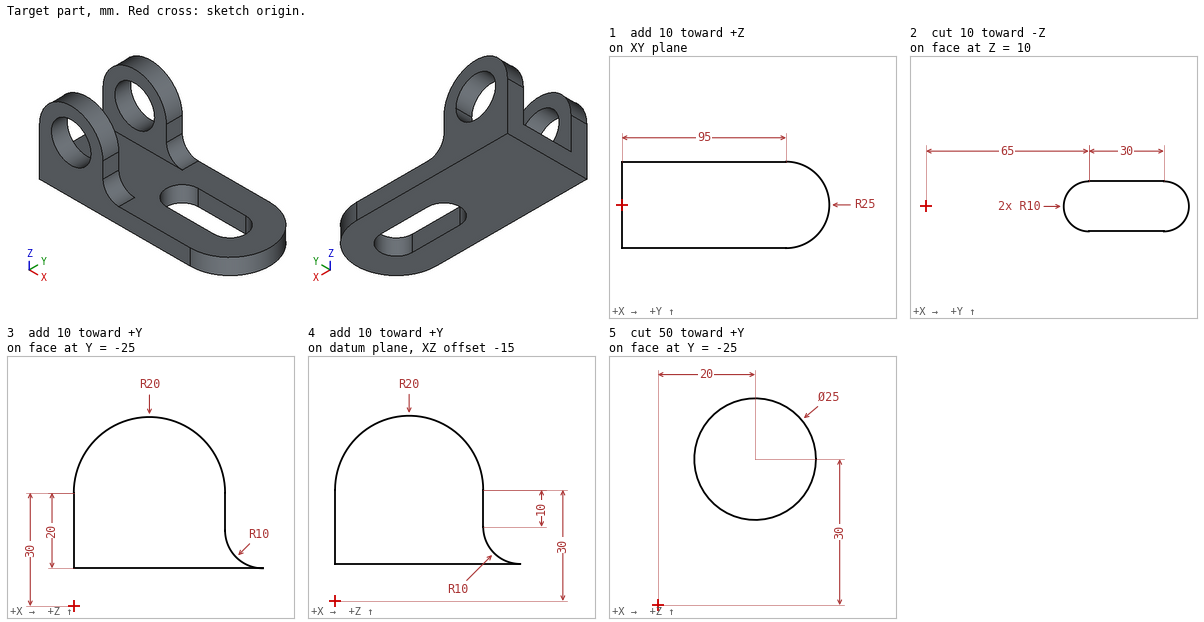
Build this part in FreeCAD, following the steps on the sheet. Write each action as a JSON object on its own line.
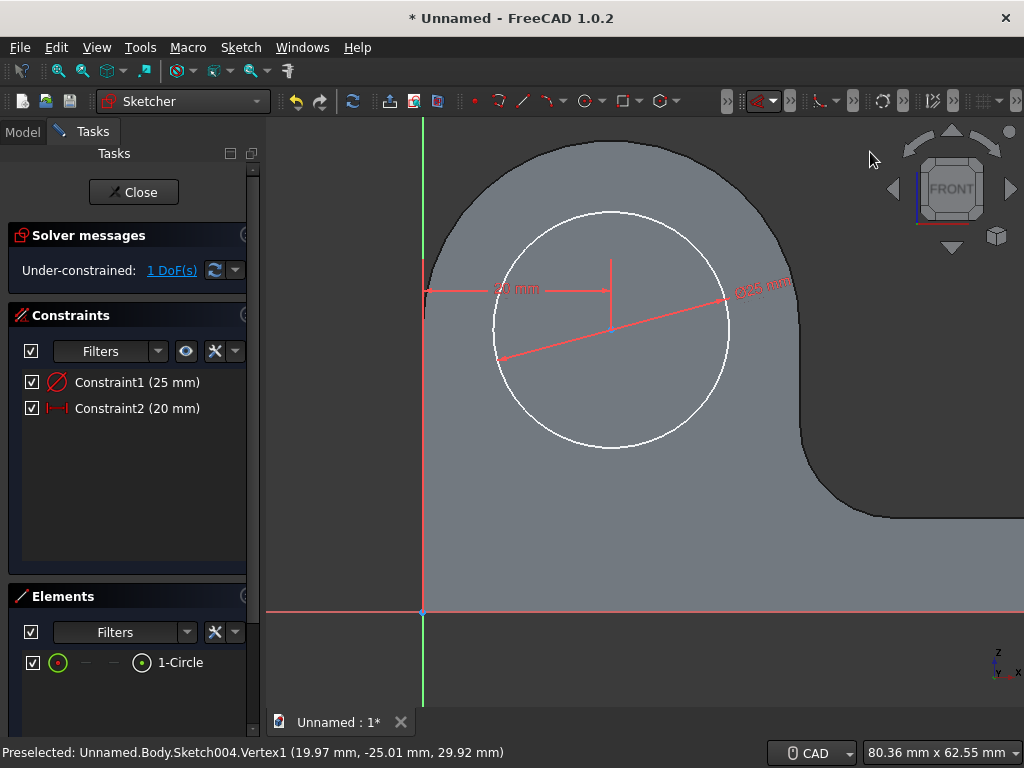
{"action": "left_click", "coordinate": [611, 330]}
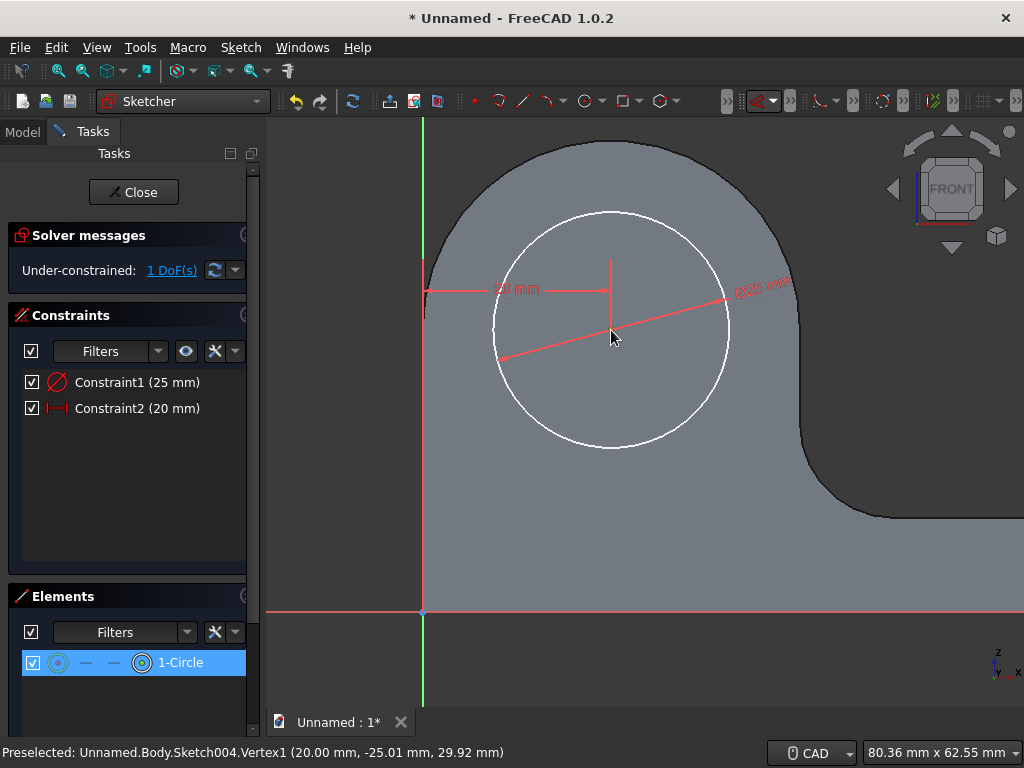
{"action": "left_click", "coordinate": [776, 102]}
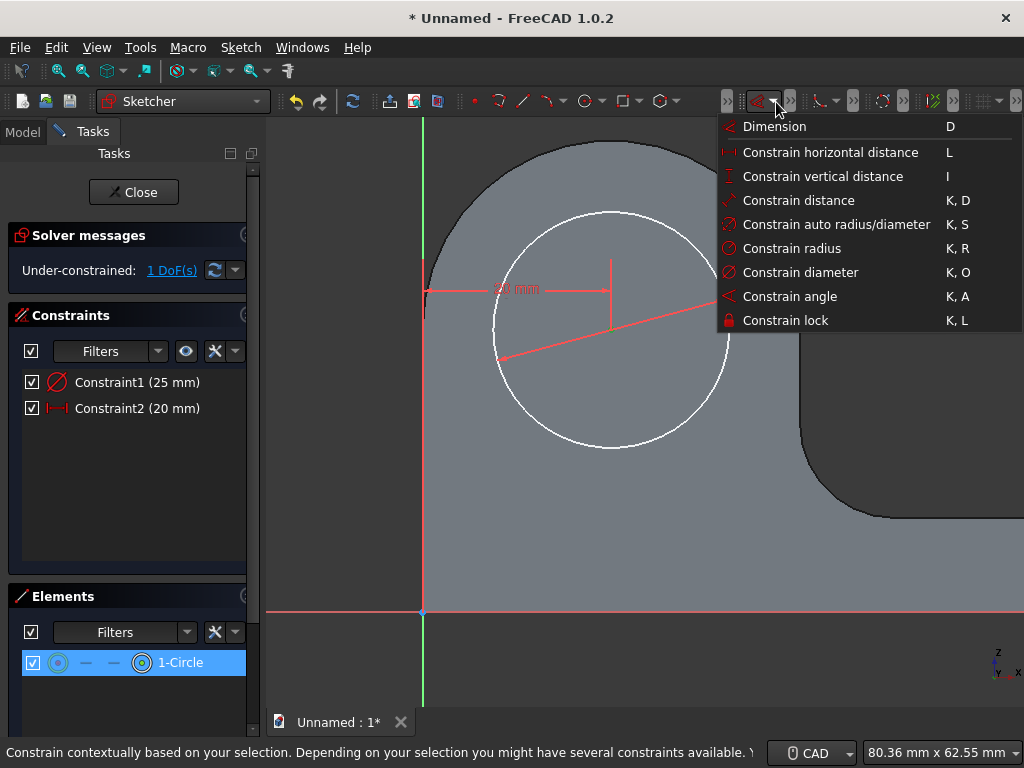
{"action": "left_click", "coordinate": [870, 176]}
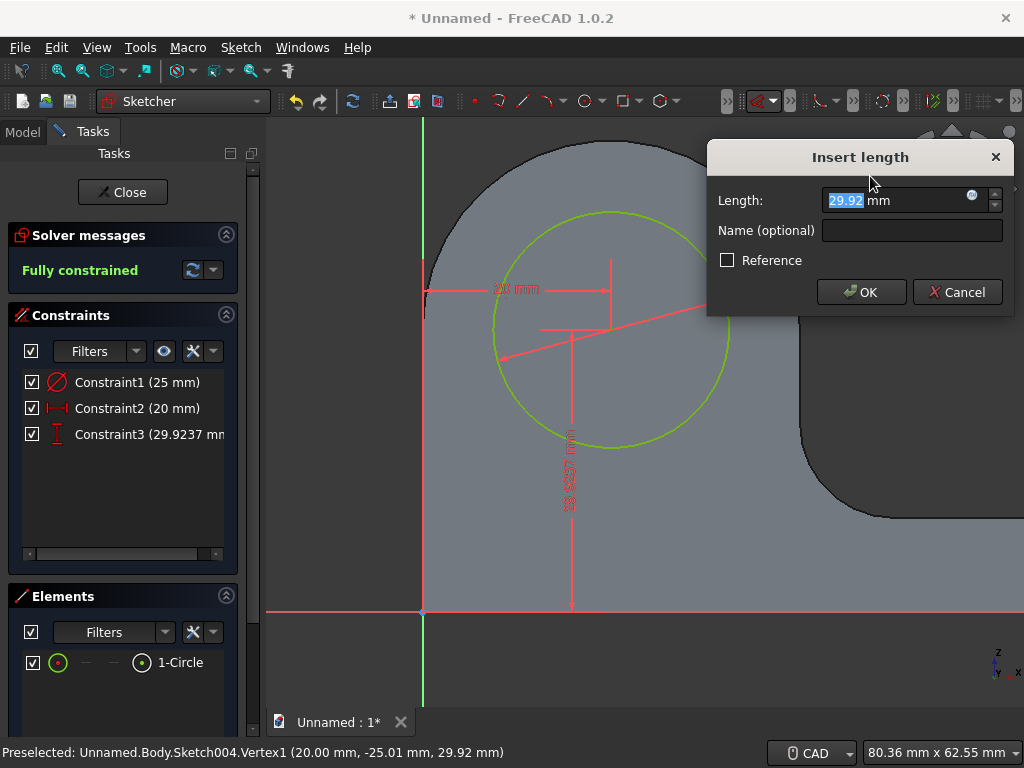
{"action": "type", "text": "30"}
{"action": "key", "text": "Return"}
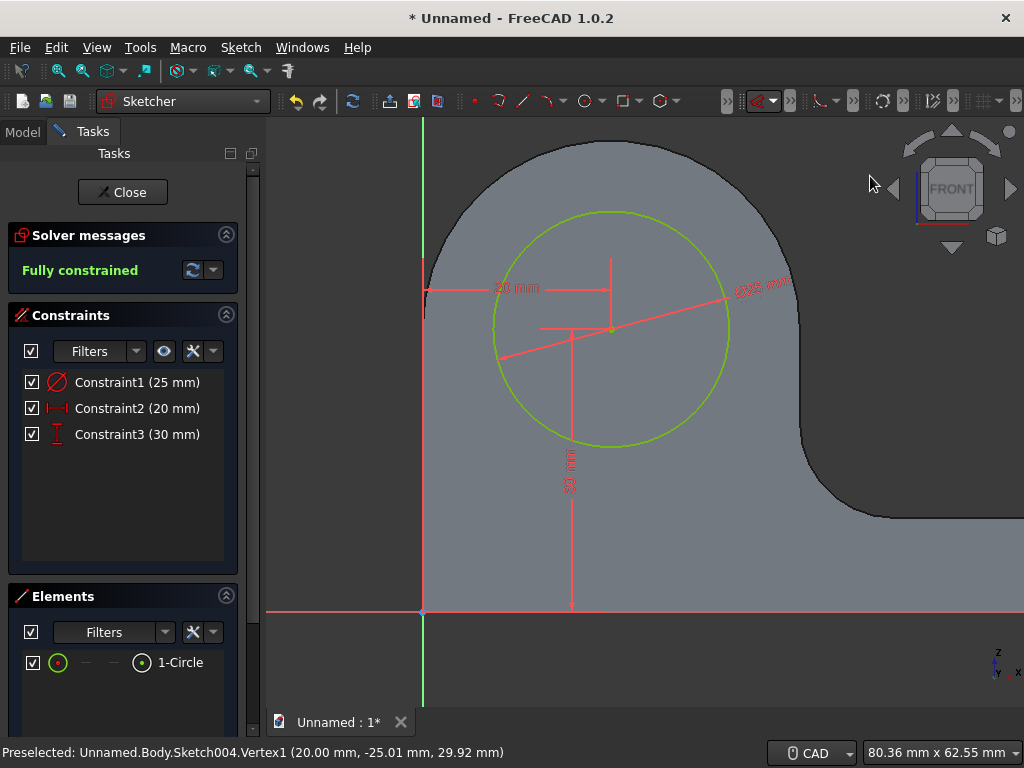
{"action": "left_click", "coordinate": [123, 192]}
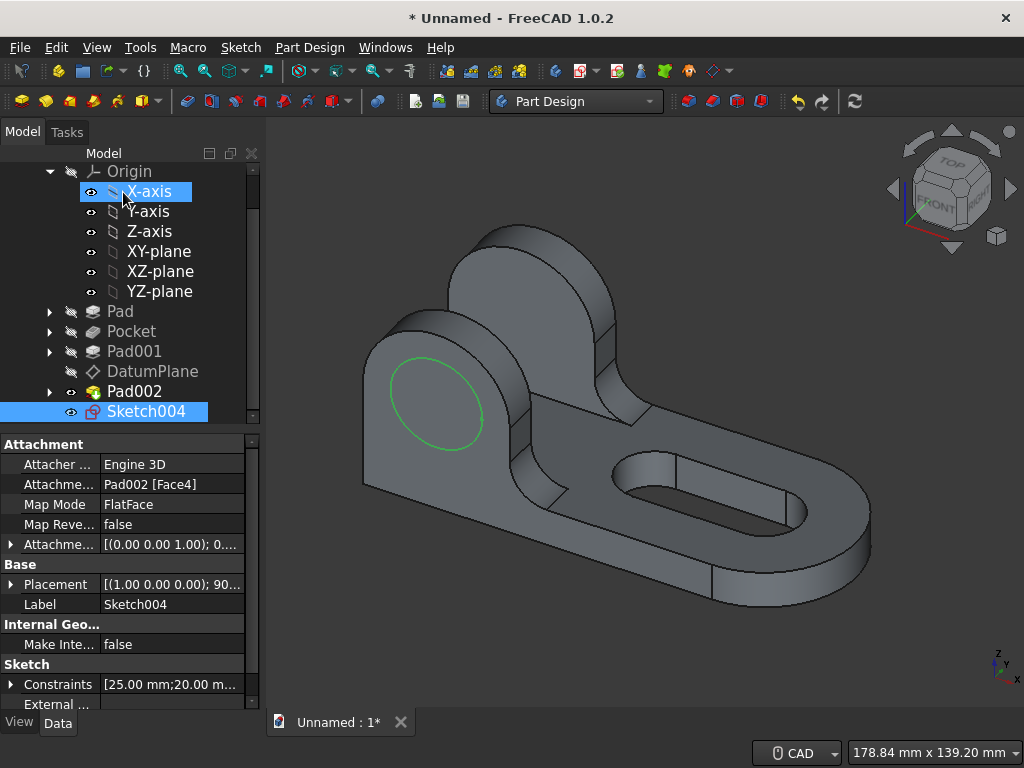
{"action": "left_click", "coordinate": [188, 102]}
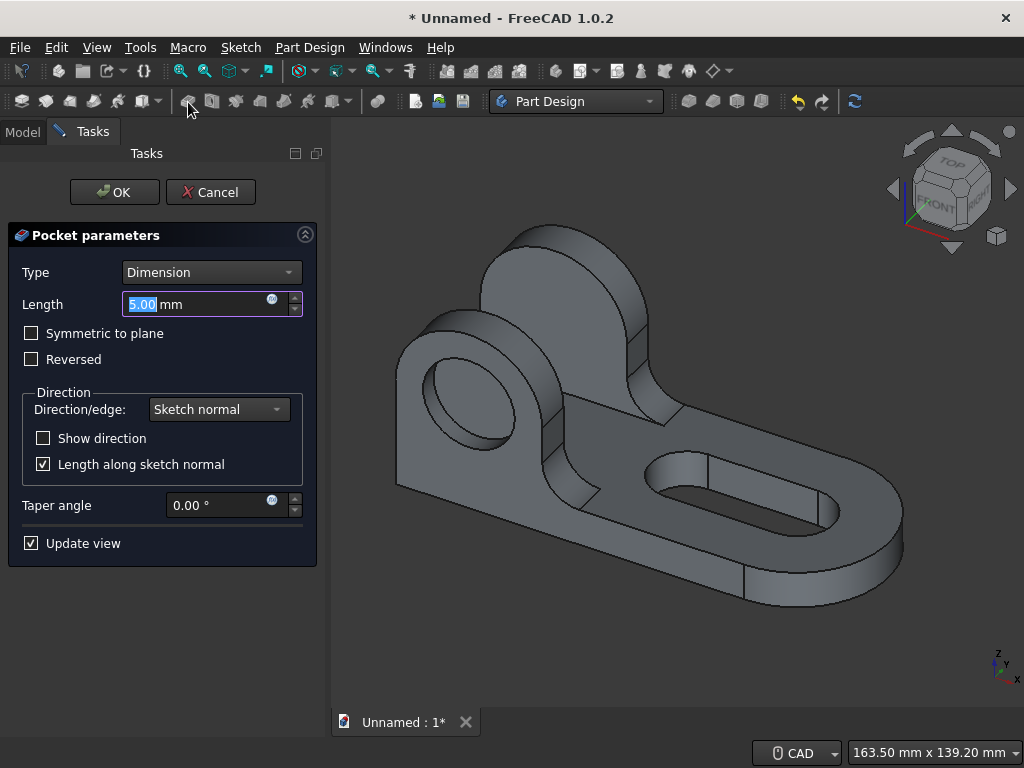
{"action": "type", "text": "50"}
{"action": "key", "text": "Tab"}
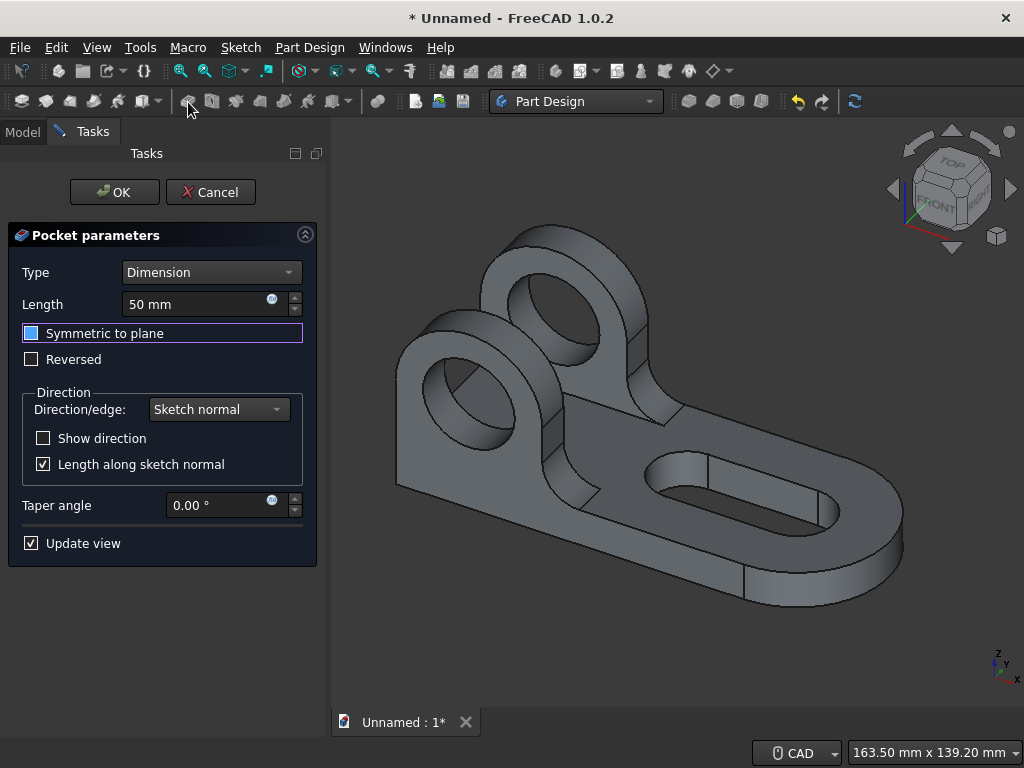
{"action": "left_click", "coordinate": [115, 192]}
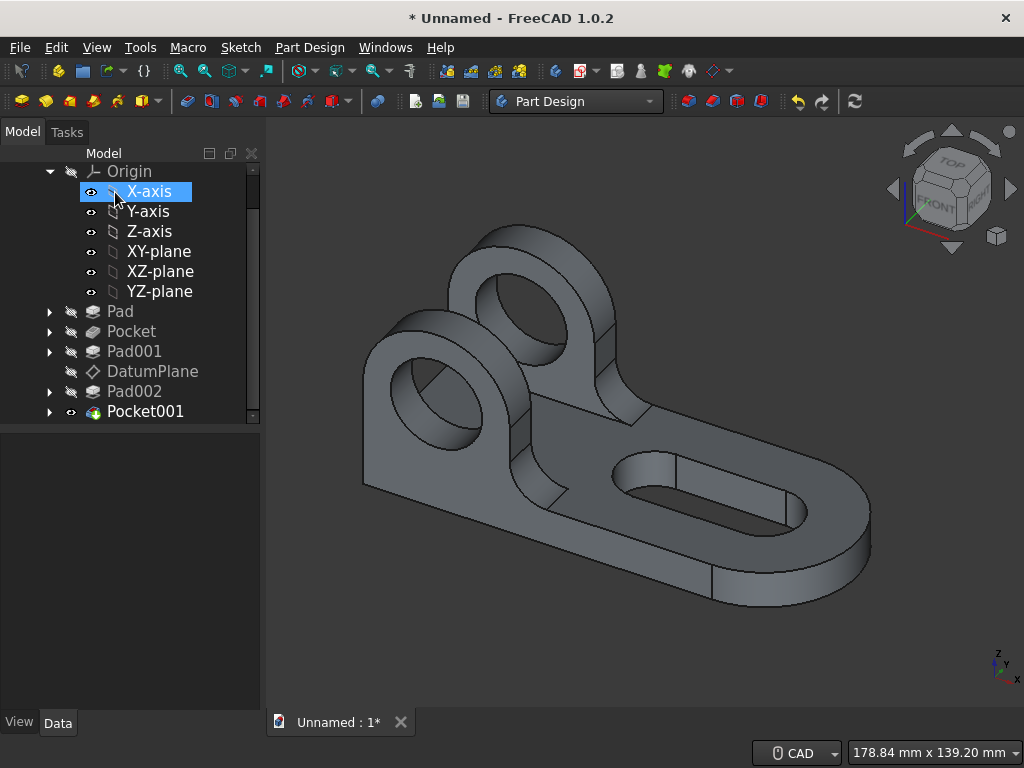
{"action": "key", "text": "0"}